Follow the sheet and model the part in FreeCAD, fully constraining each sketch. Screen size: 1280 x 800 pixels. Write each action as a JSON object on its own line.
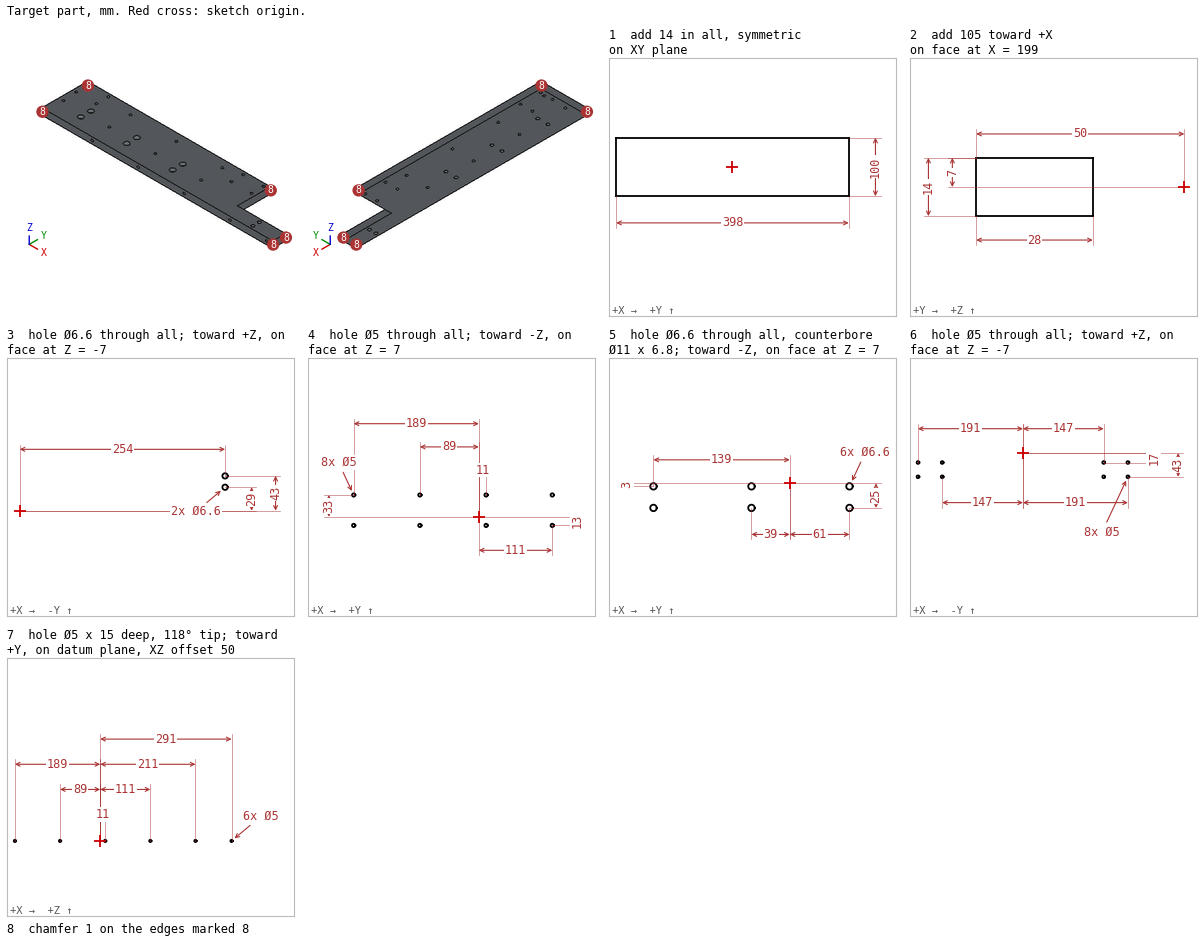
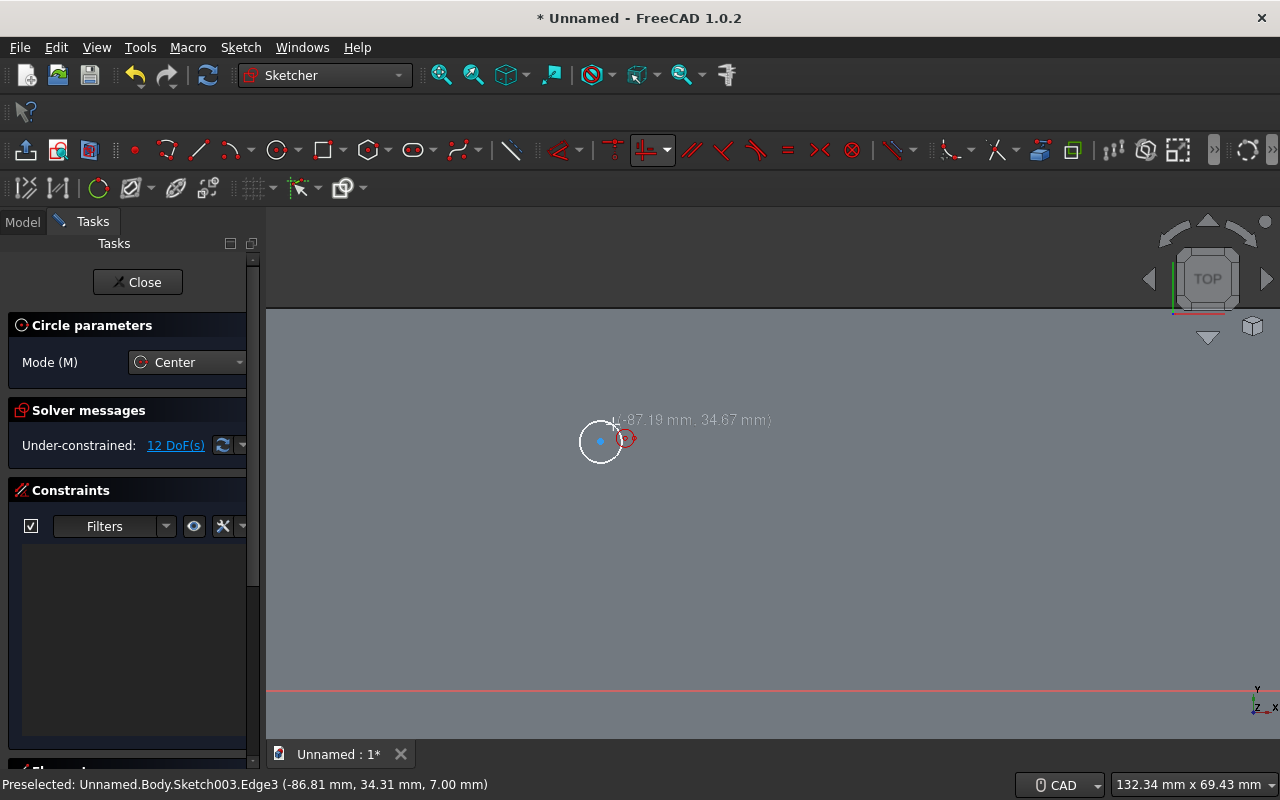
{"action": "scroll", "coordinate": [614, 427], "scroll_direction": "down", "scroll_amount": 7}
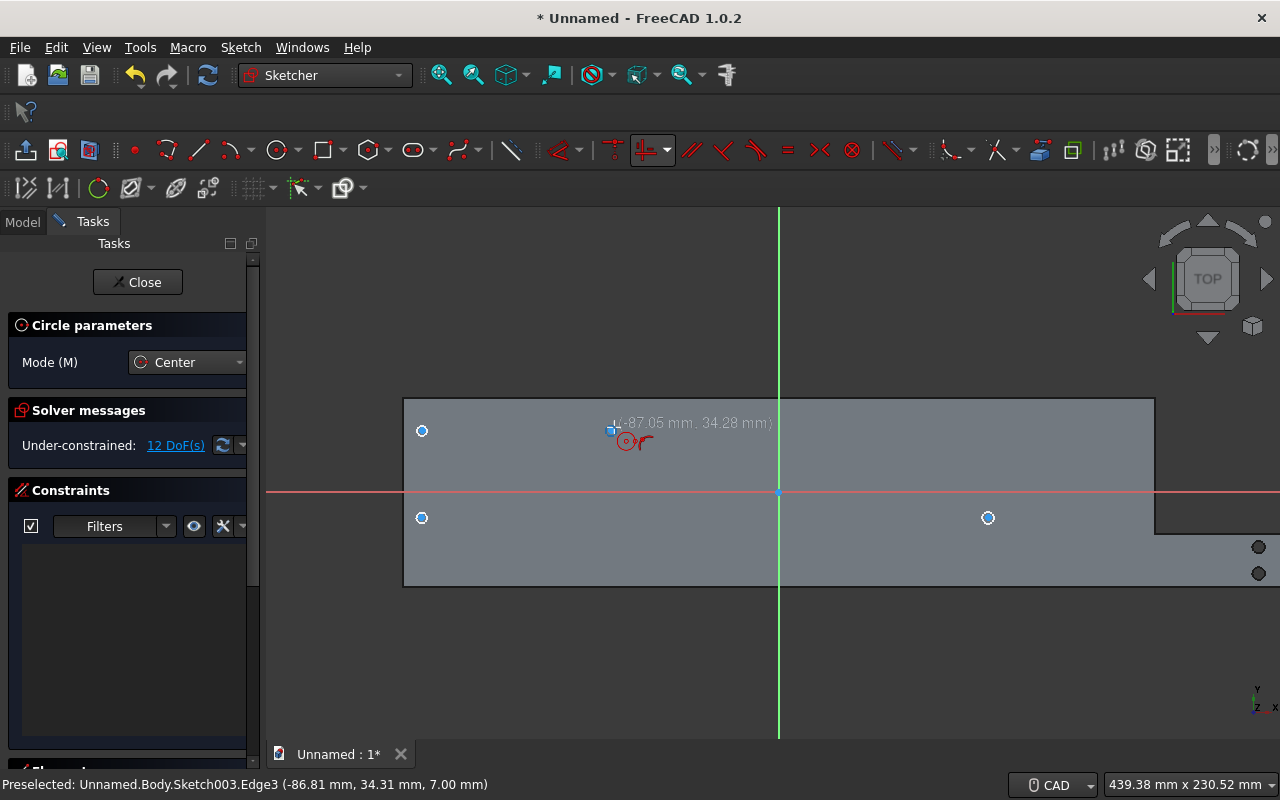
{"action": "scroll", "coordinate": [611, 517], "scroll_direction": "up", "scroll_amount": 8}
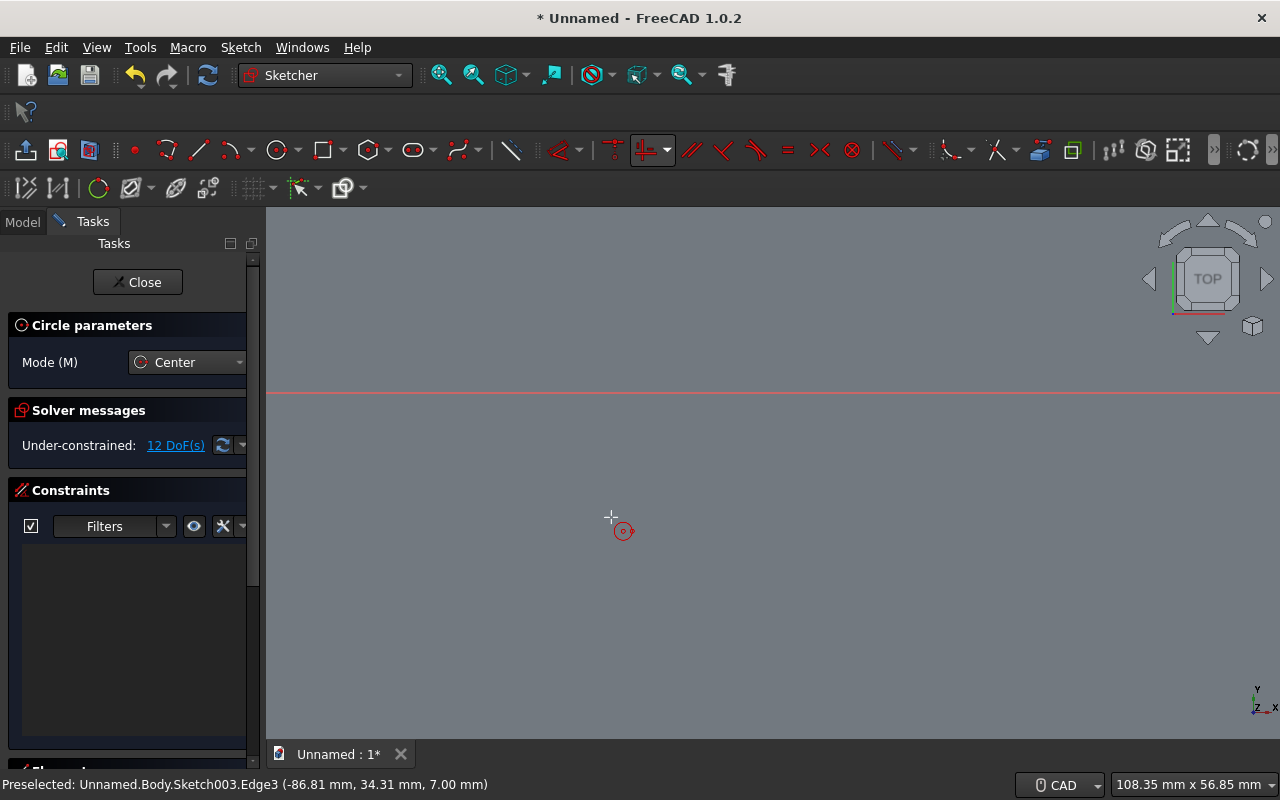
{"action": "scroll", "coordinate": [611, 517], "scroll_direction": "down", "scroll_amount": 8}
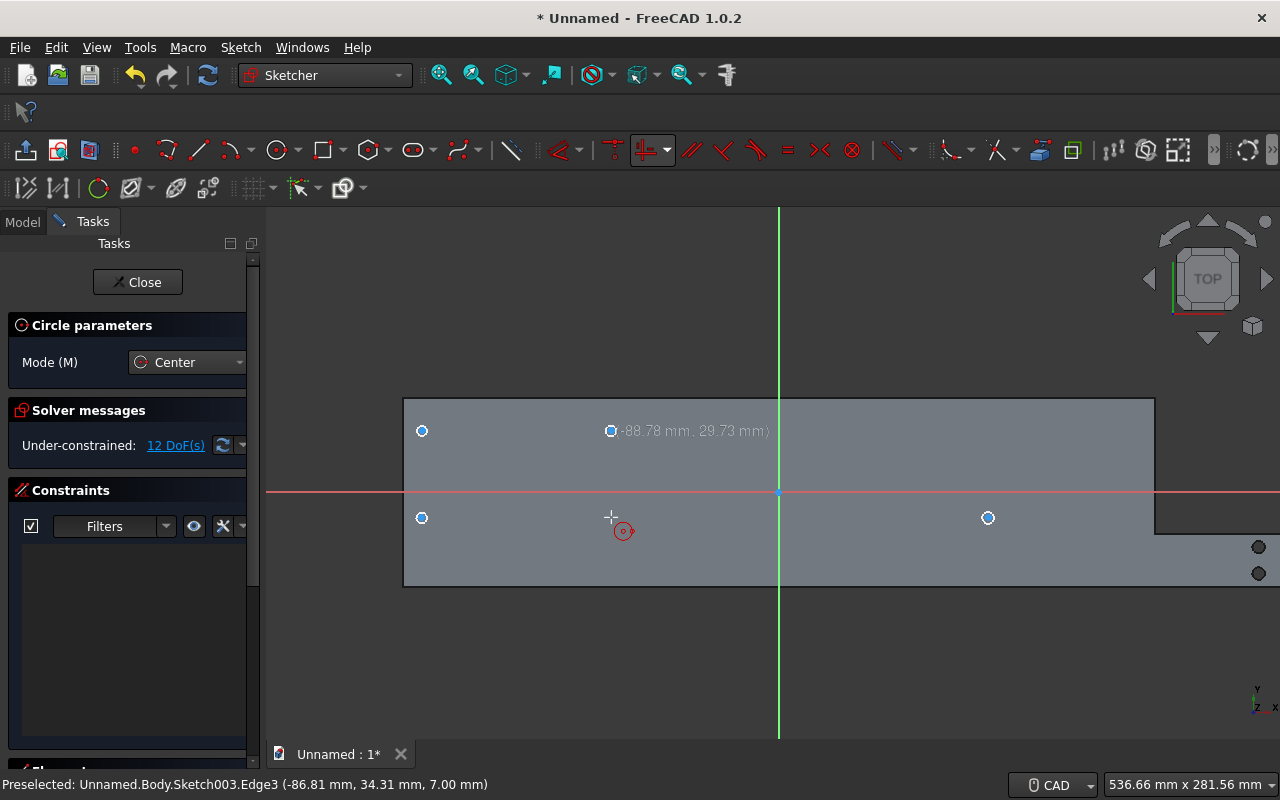
{"action": "left_click", "coordinate": [611, 517]}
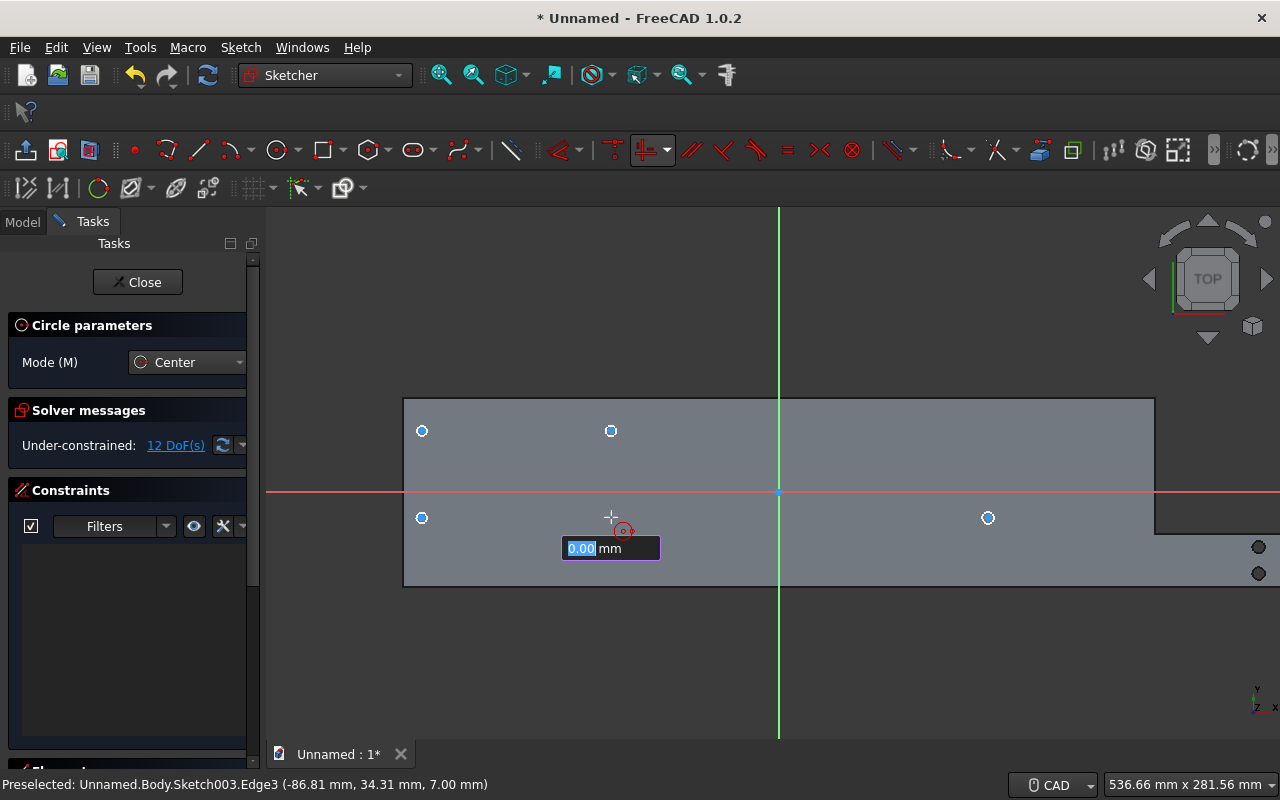
{"action": "scroll", "coordinate": [614, 514], "scroll_direction": "up", "scroll_amount": 7}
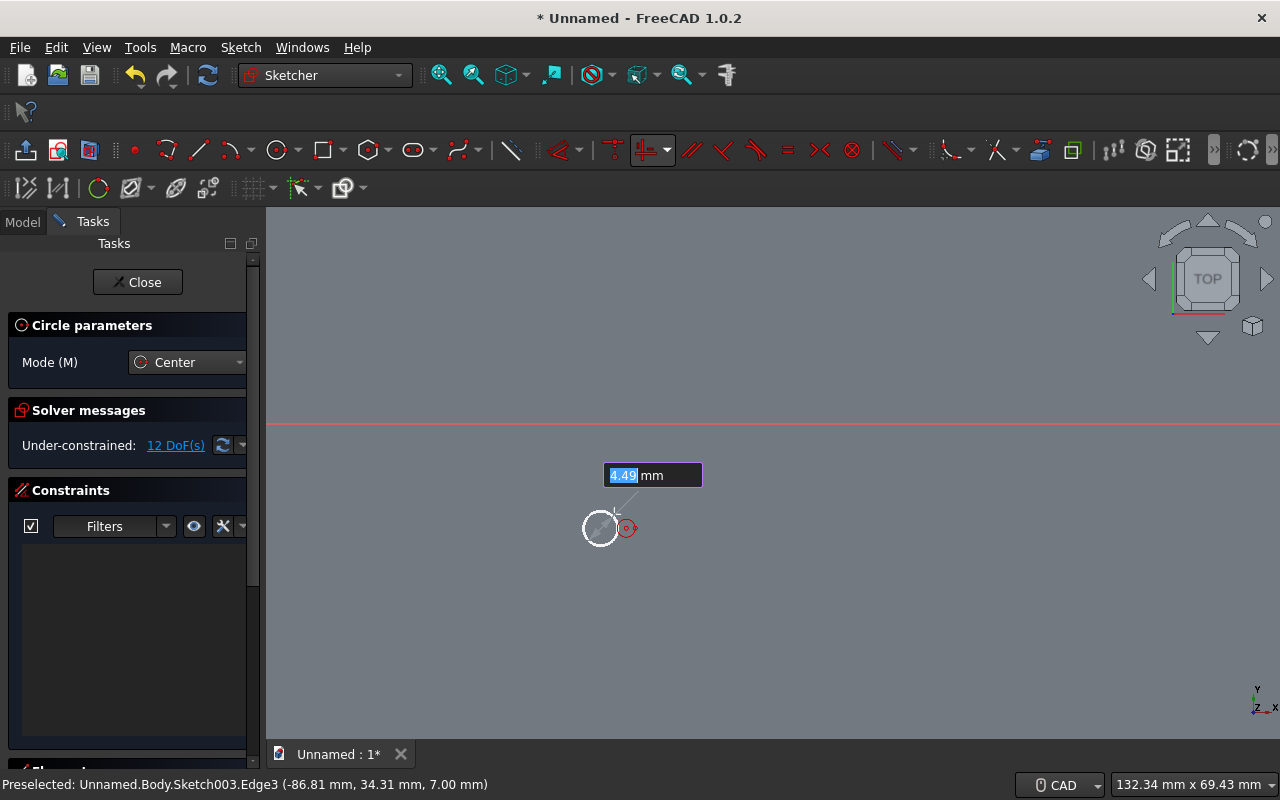
{"action": "left_click", "coordinate": [613, 510]}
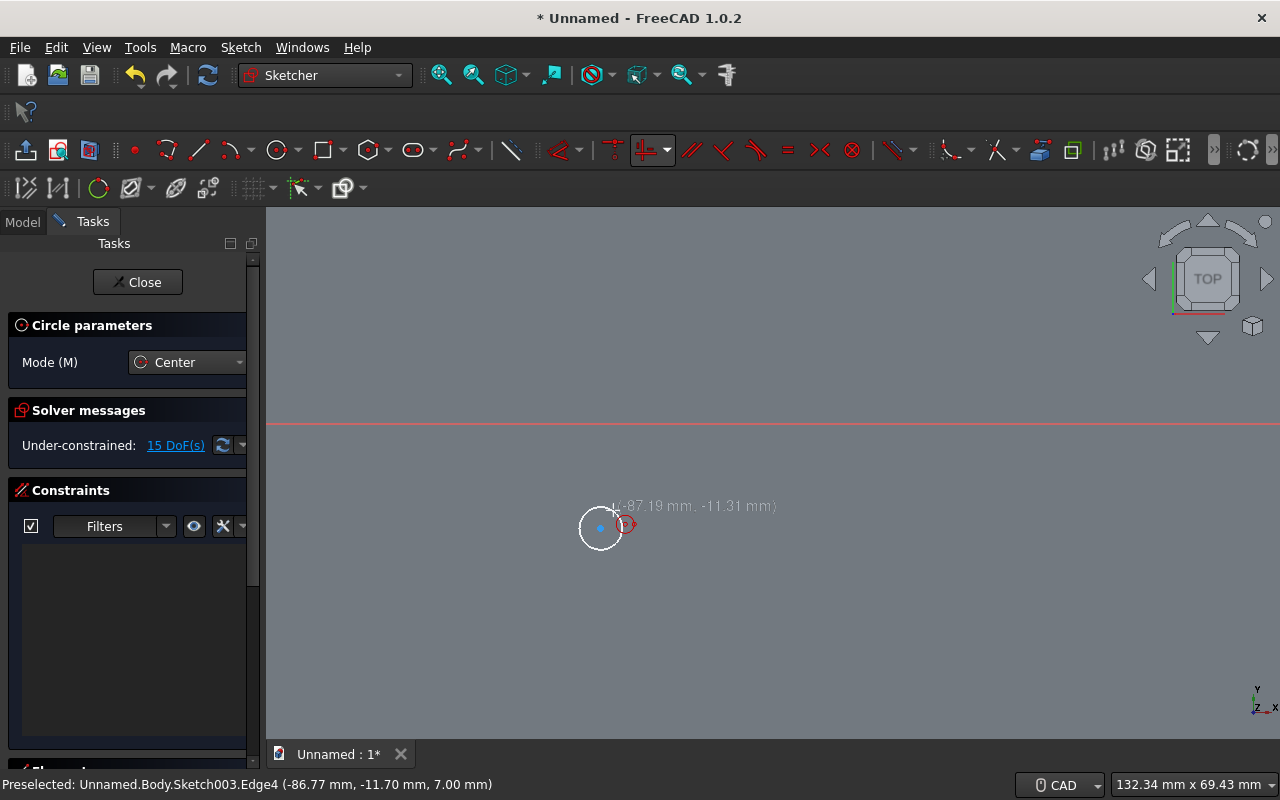
{"action": "scroll", "coordinate": [614, 514], "scroll_direction": "down", "scroll_amount": 7}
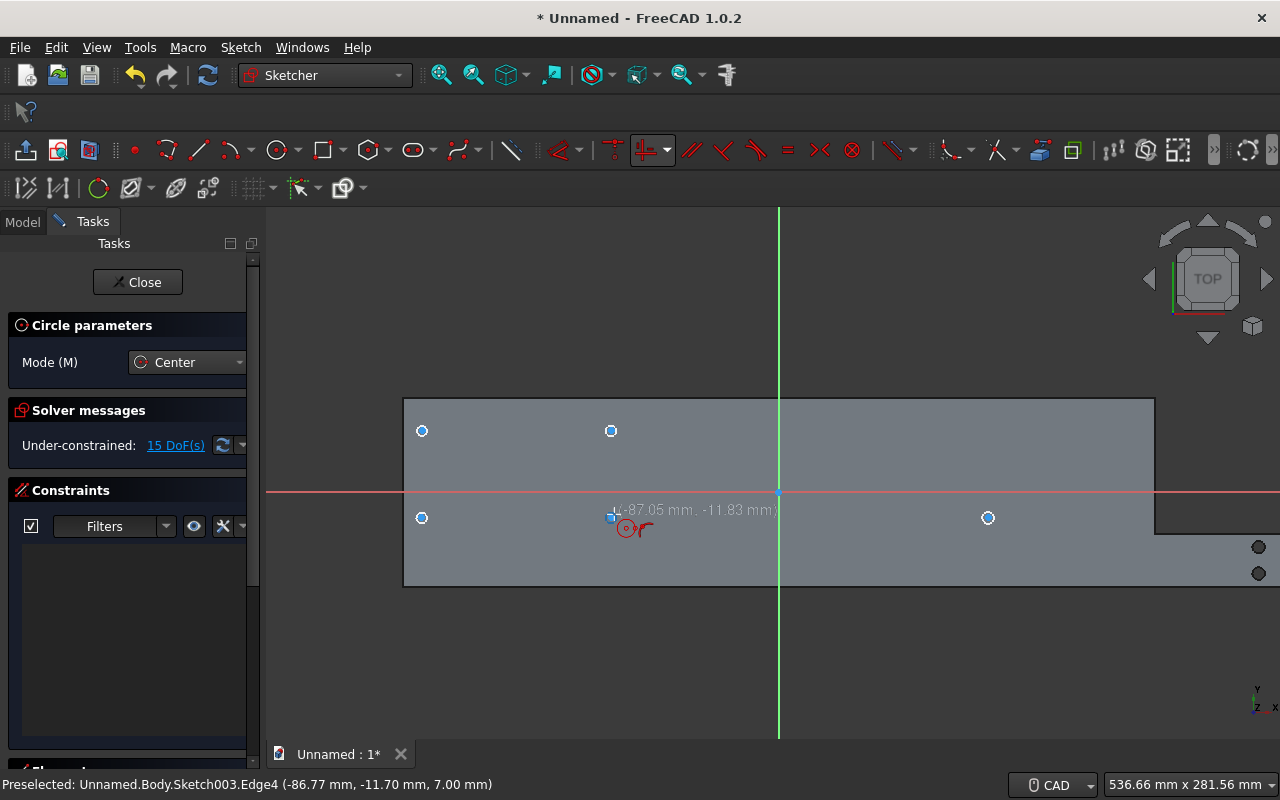
{"action": "scroll", "coordinate": [800, 430], "scroll_direction": "up", "scroll_amount": 8}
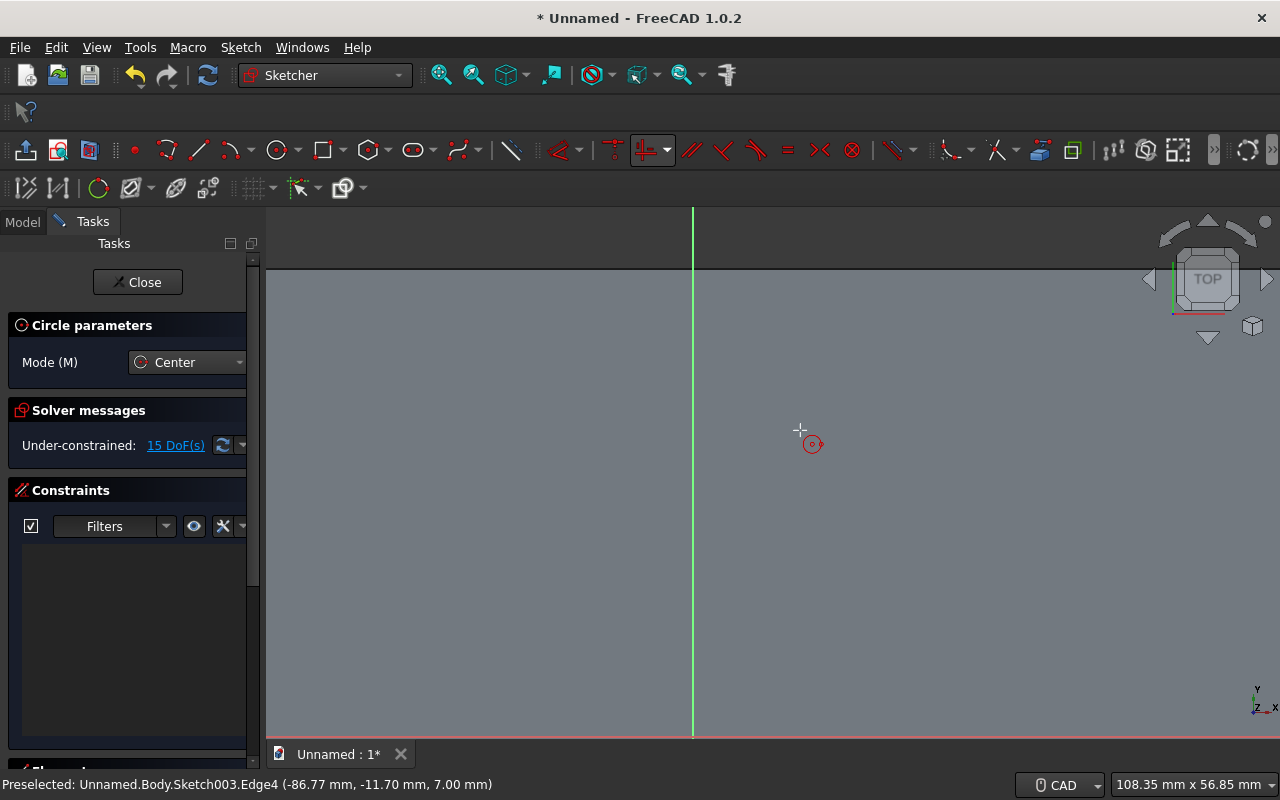
{"action": "scroll", "coordinate": [800, 430], "scroll_direction": "down", "scroll_amount": 8}